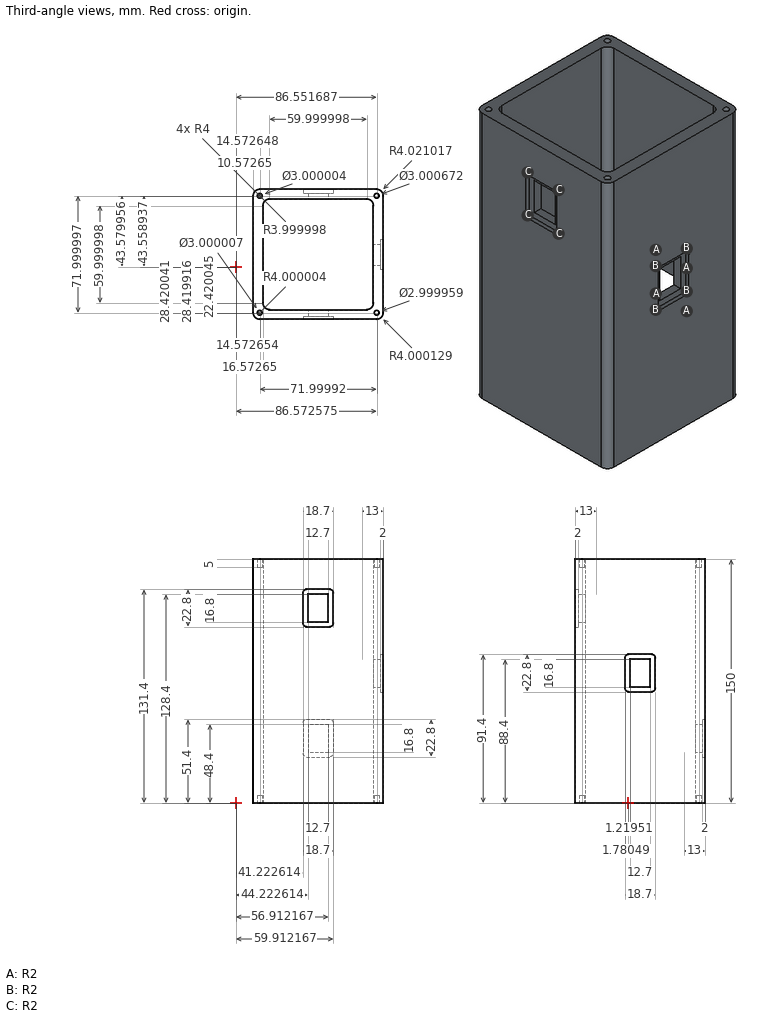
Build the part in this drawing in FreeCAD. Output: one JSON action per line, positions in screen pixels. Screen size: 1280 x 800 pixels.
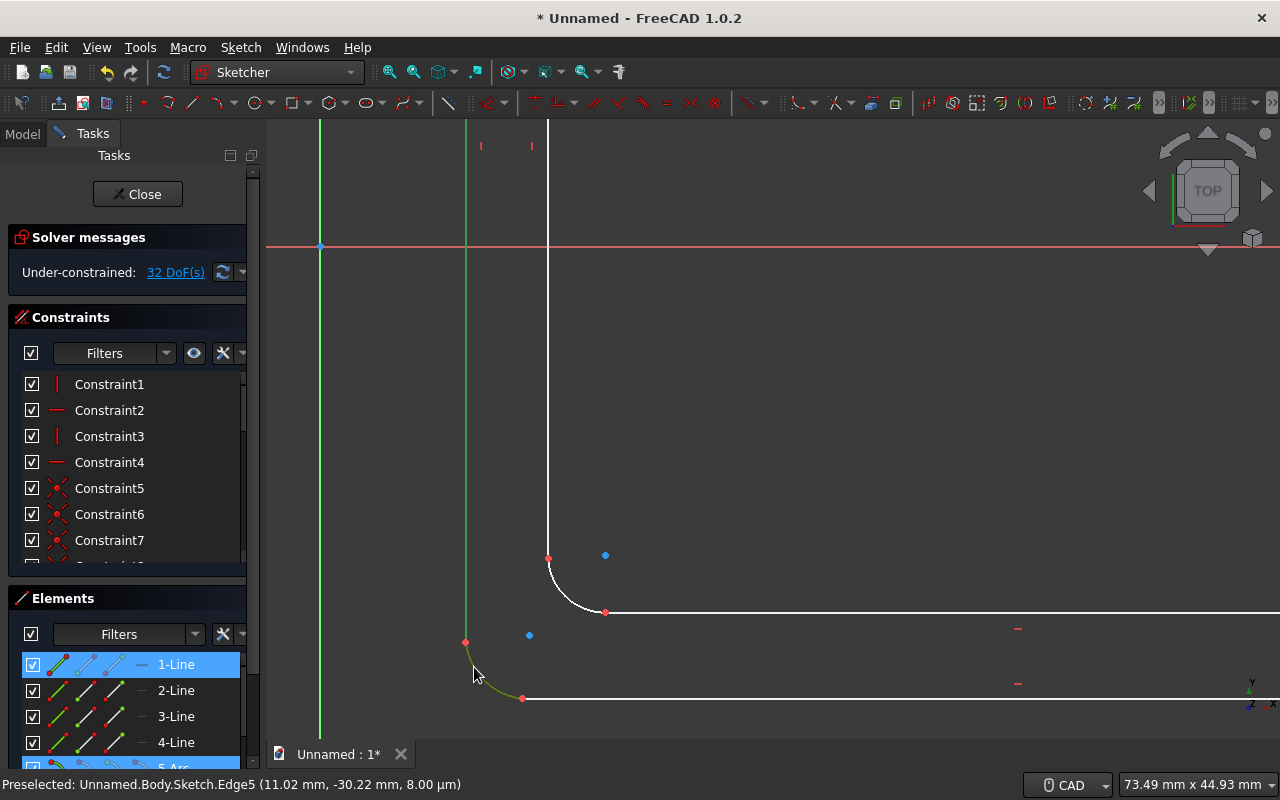
{"action": "left_click", "coordinate": [644, 104]}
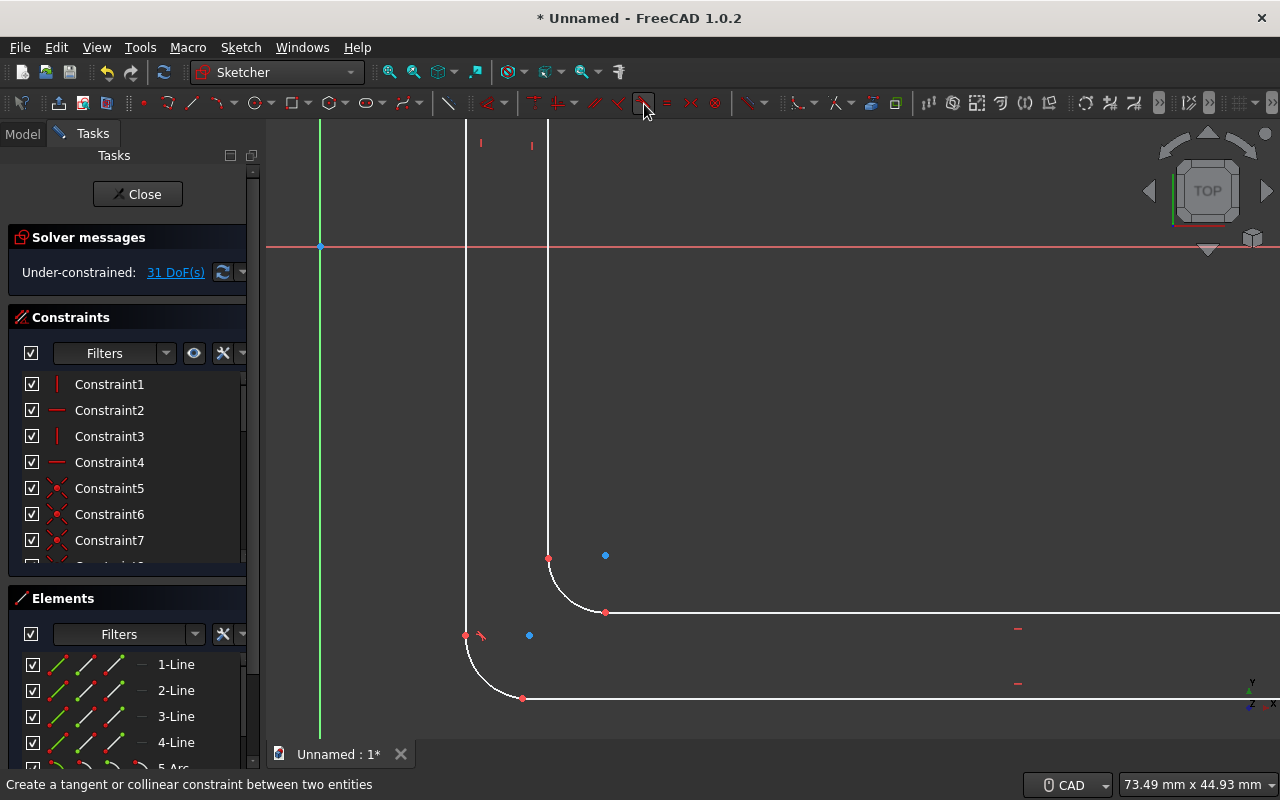
{"action": "left_click", "coordinate": [466, 340]}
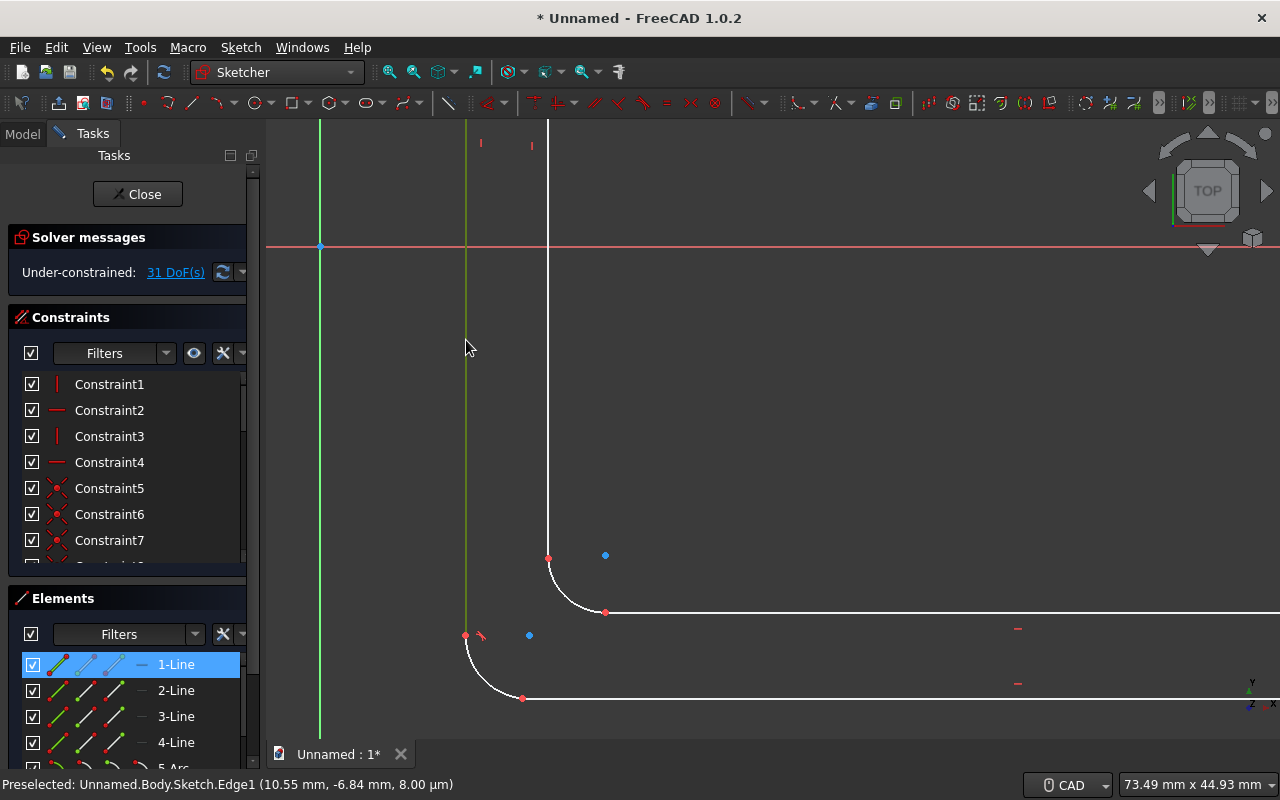
{"action": "scroll", "coordinate": [565, 596], "scroll_direction": "down", "scroll_amount": 5}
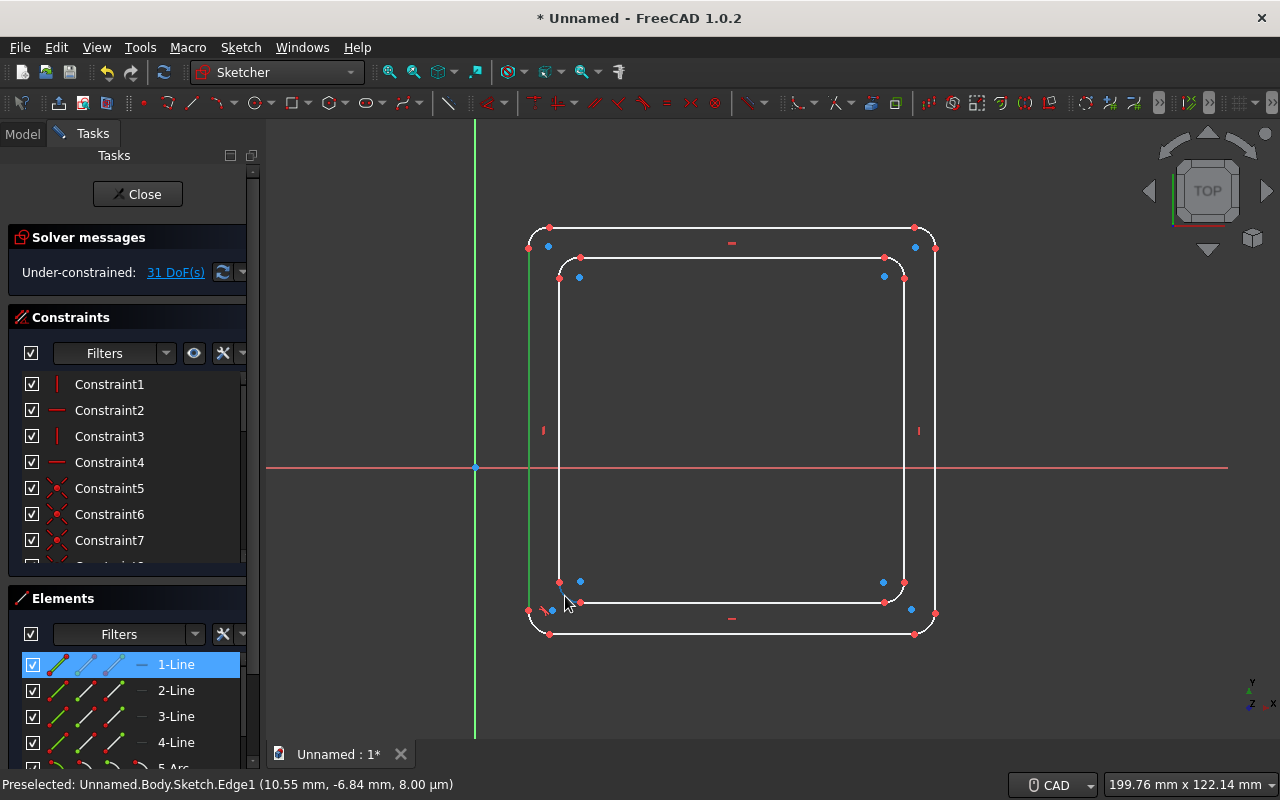
{"action": "scroll", "coordinate": [540, 229], "scroll_direction": "up", "scroll_amount": 2}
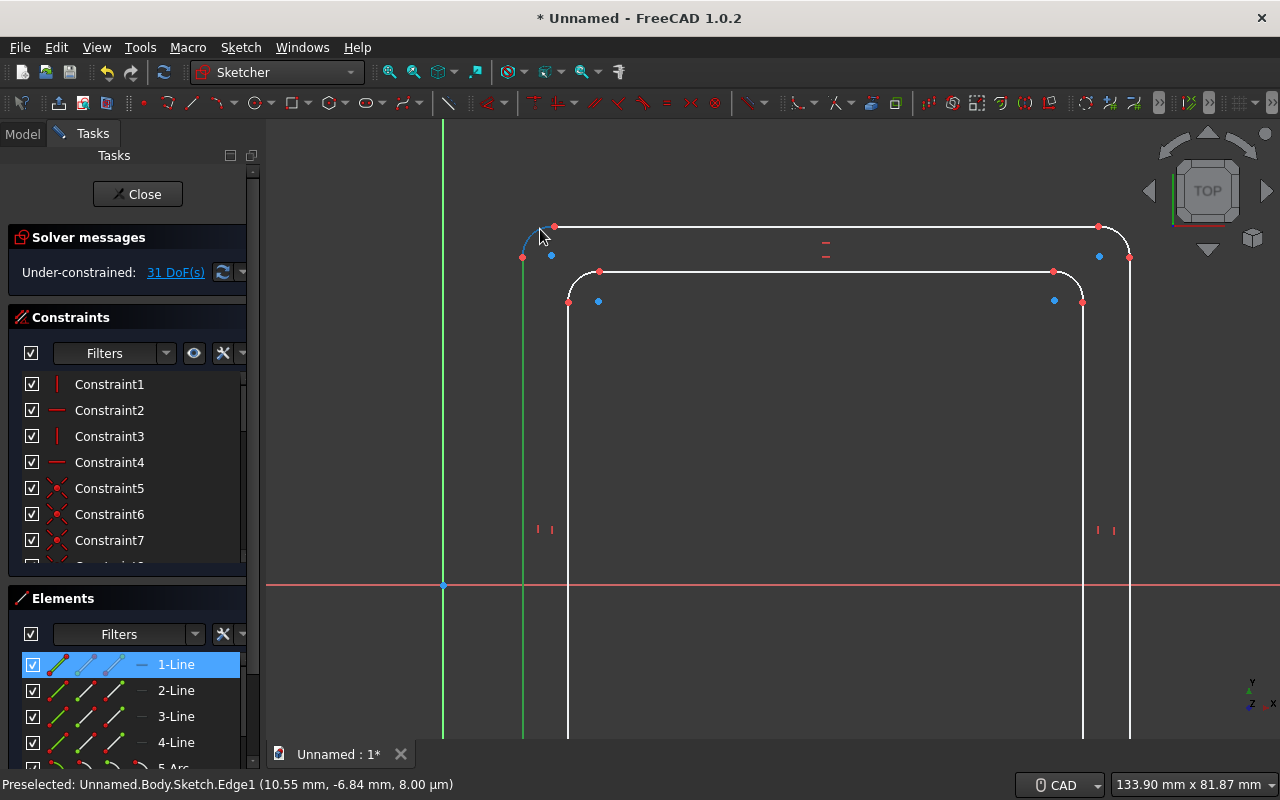
{"action": "left_click", "coordinate": [540, 229]}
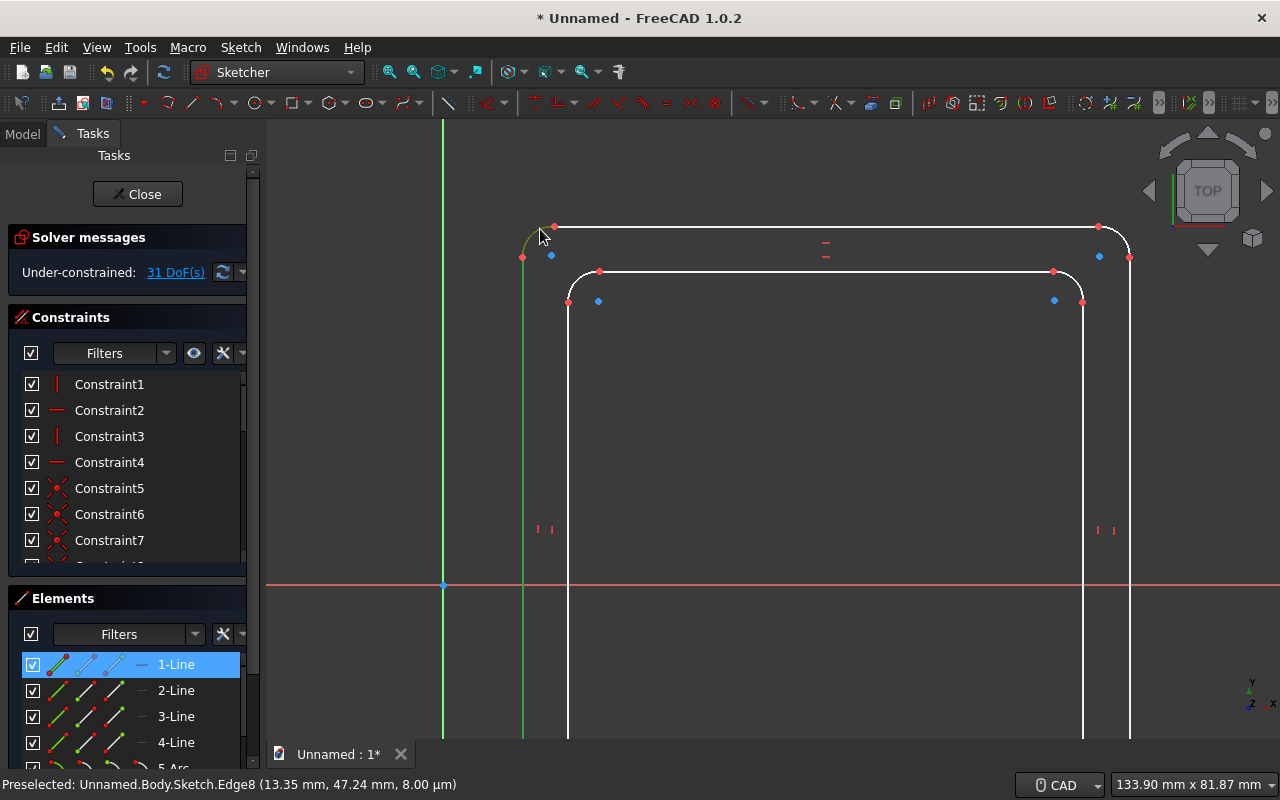
{"action": "key", "text": "t"}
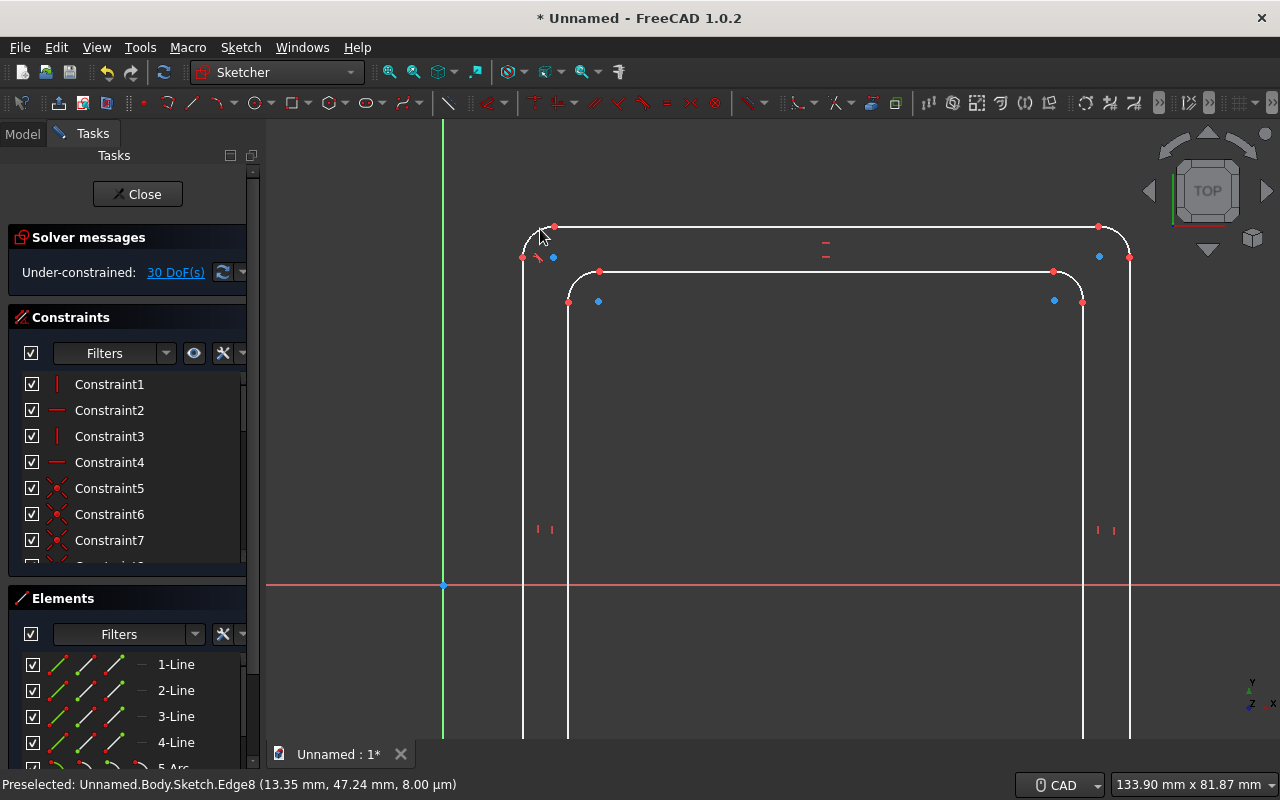
{"action": "scroll", "coordinate": [539, 228], "scroll_direction": "down", "scroll_amount": 2}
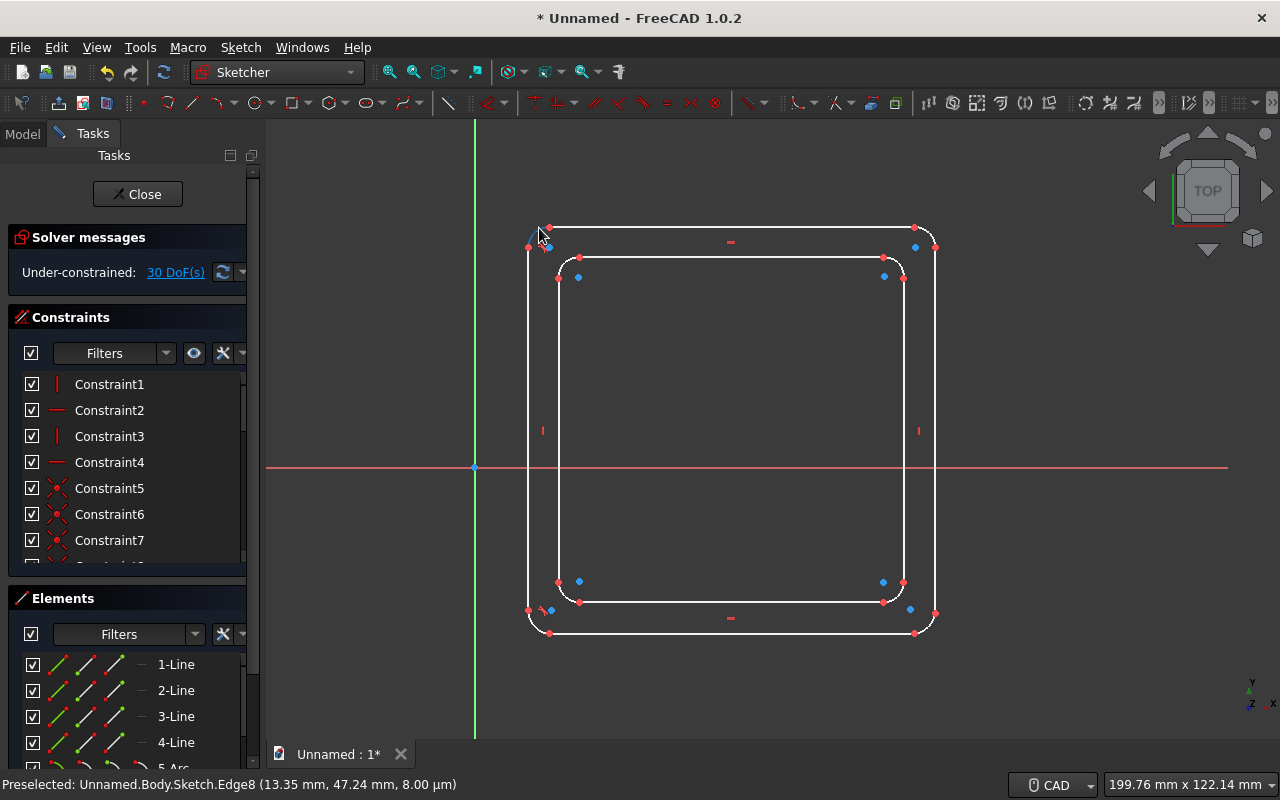
{"action": "left_click", "coordinate": [659, 634]}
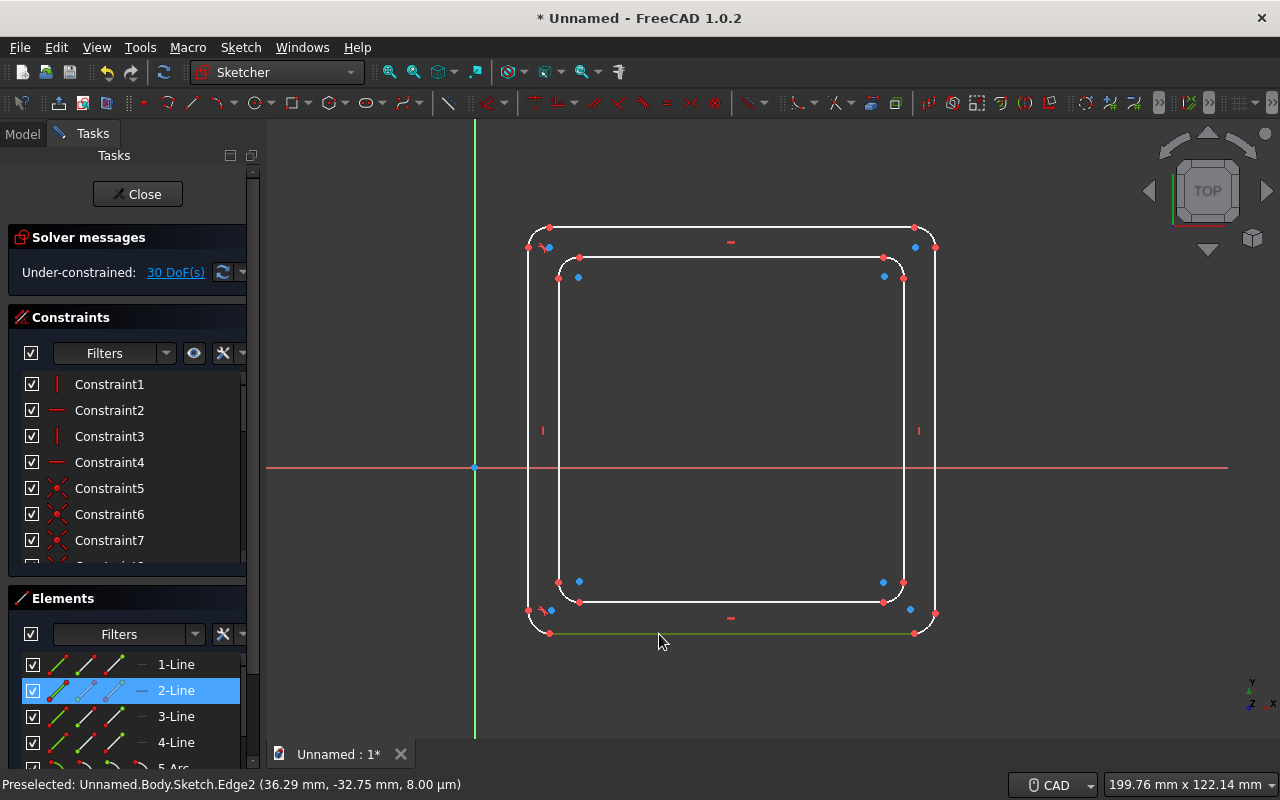
{"action": "scroll", "coordinate": [531, 621], "scroll_direction": "up", "scroll_amount": 2}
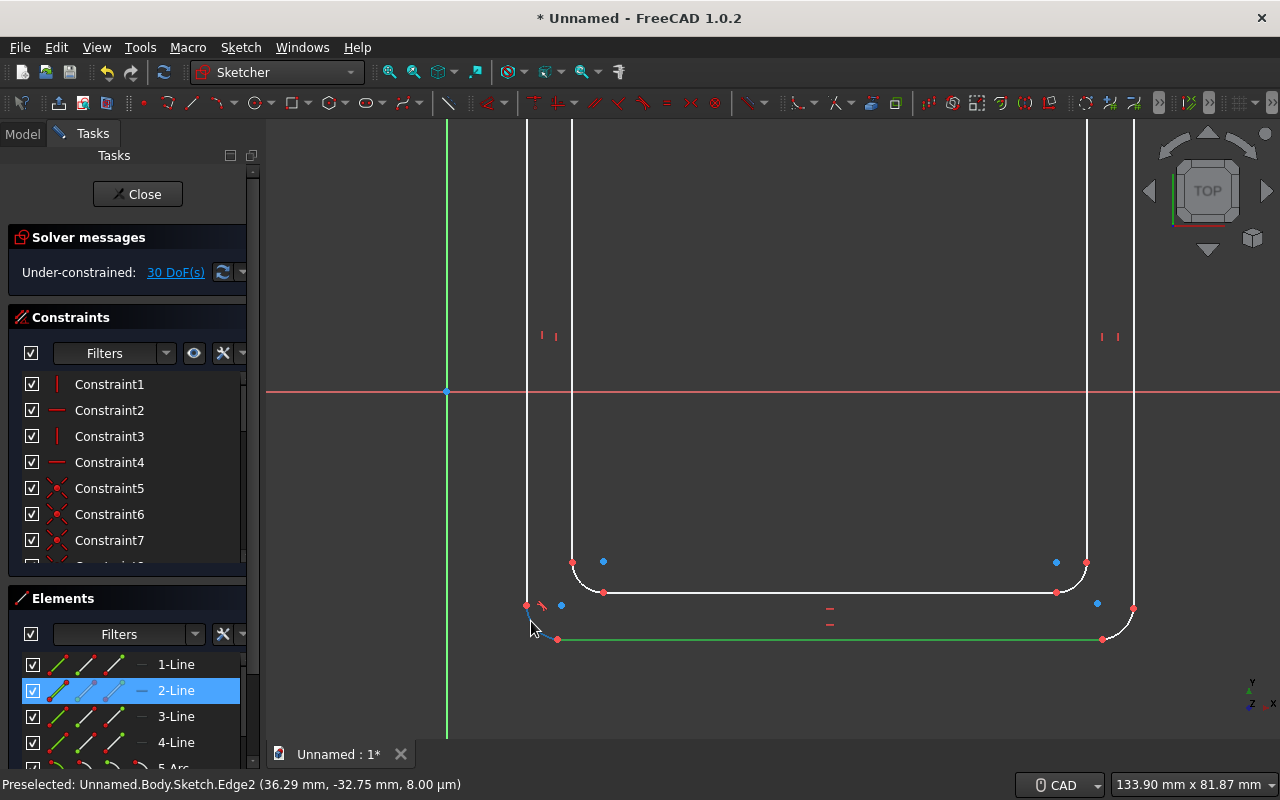
{"action": "left_click", "coordinate": [530, 620]}